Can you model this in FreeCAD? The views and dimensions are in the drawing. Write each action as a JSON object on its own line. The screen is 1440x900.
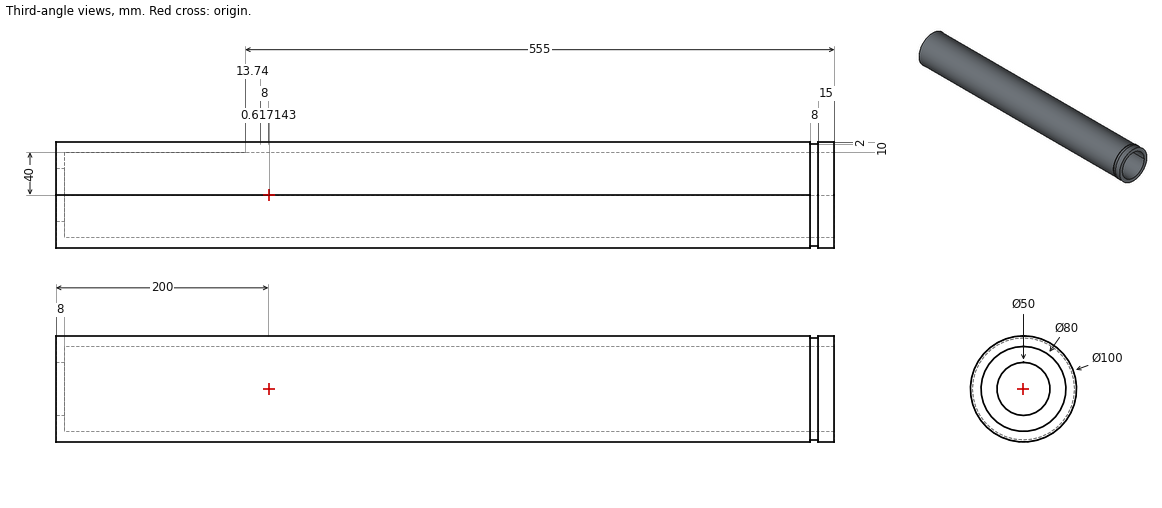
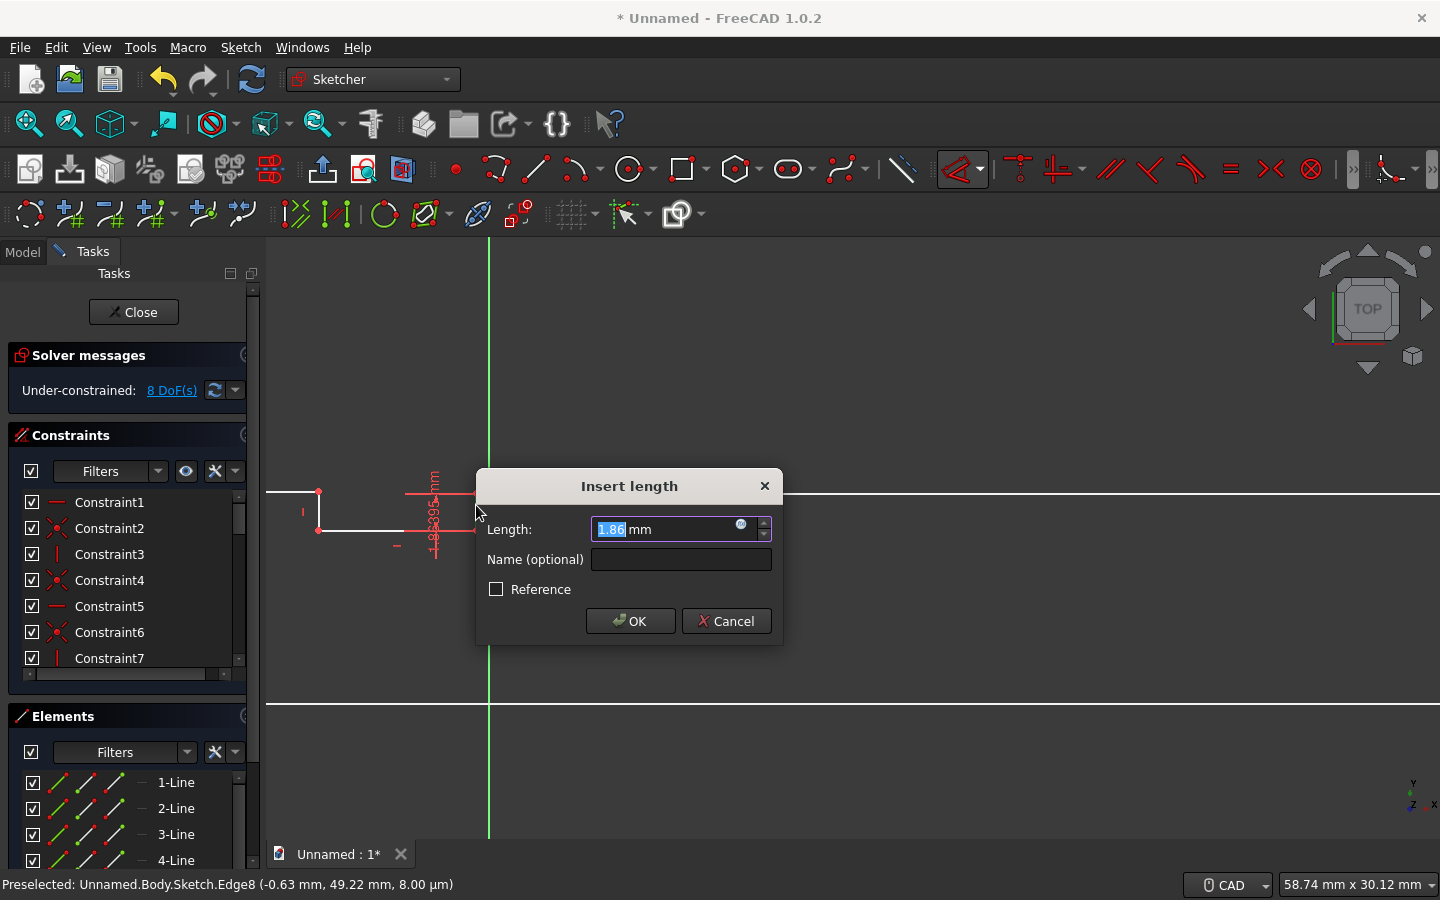
{"action": "type", "text": "2"}
{"action": "key", "text": "Return"}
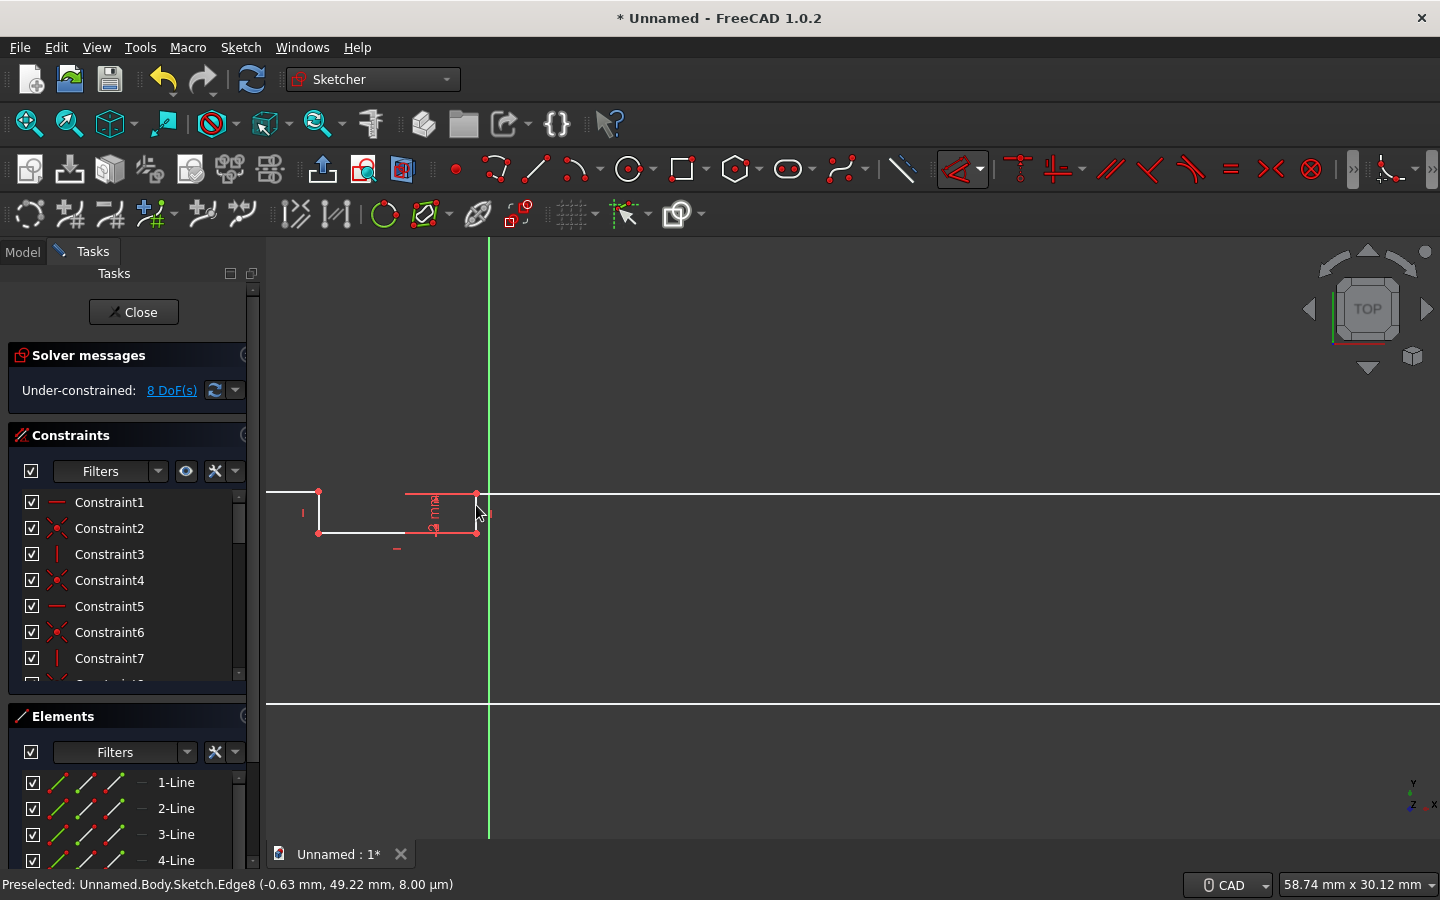
{"action": "scroll", "coordinate": [473, 509], "scroll_direction": "down", "scroll_amount": 14}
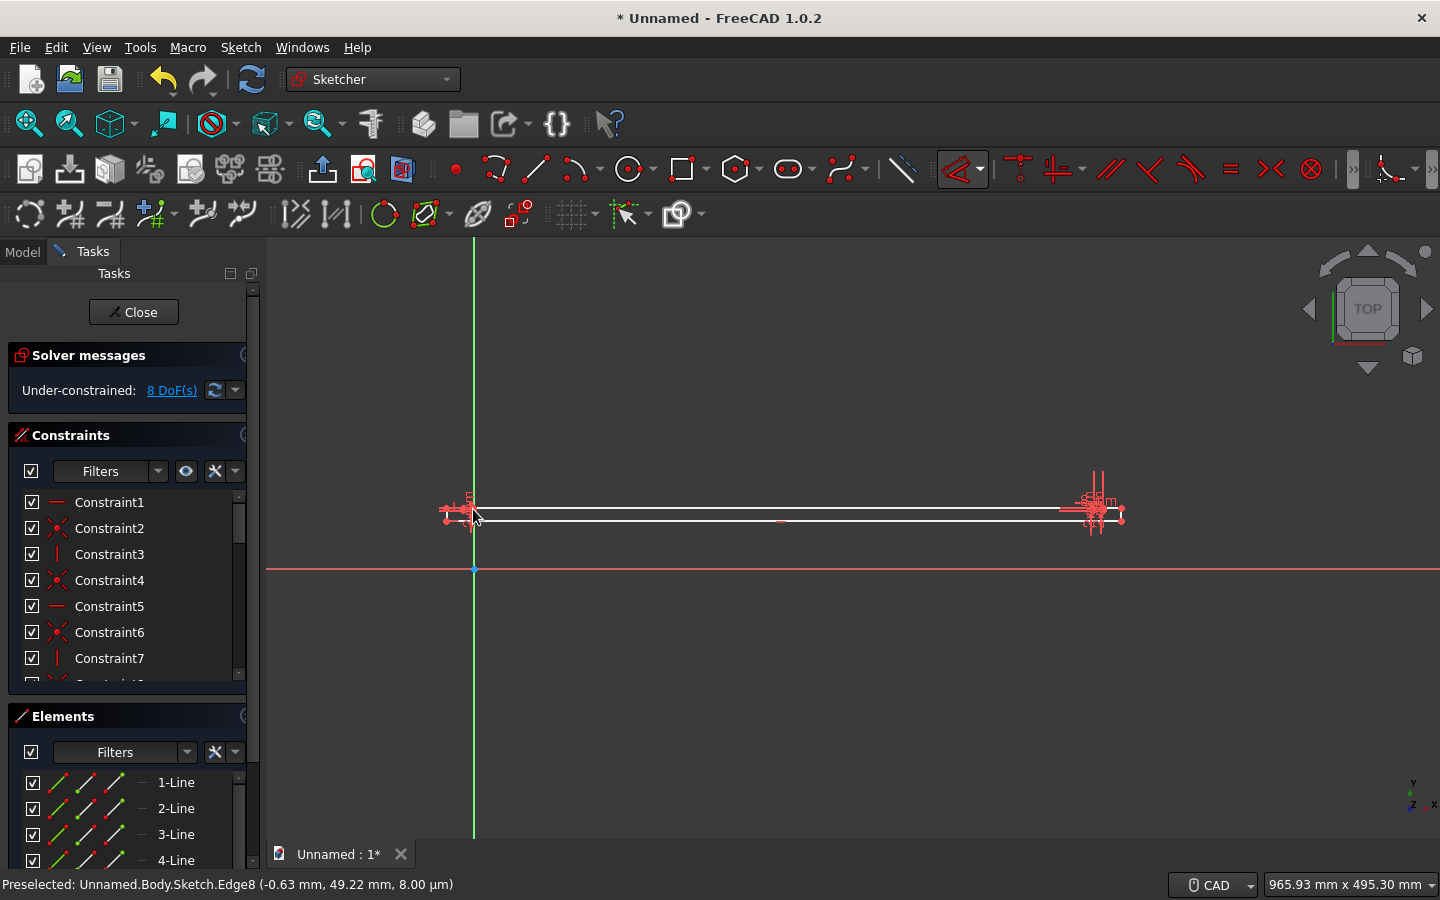
{"action": "scroll", "coordinate": [470, 511], "scroll_direction": "up", "scroll_amount": 8}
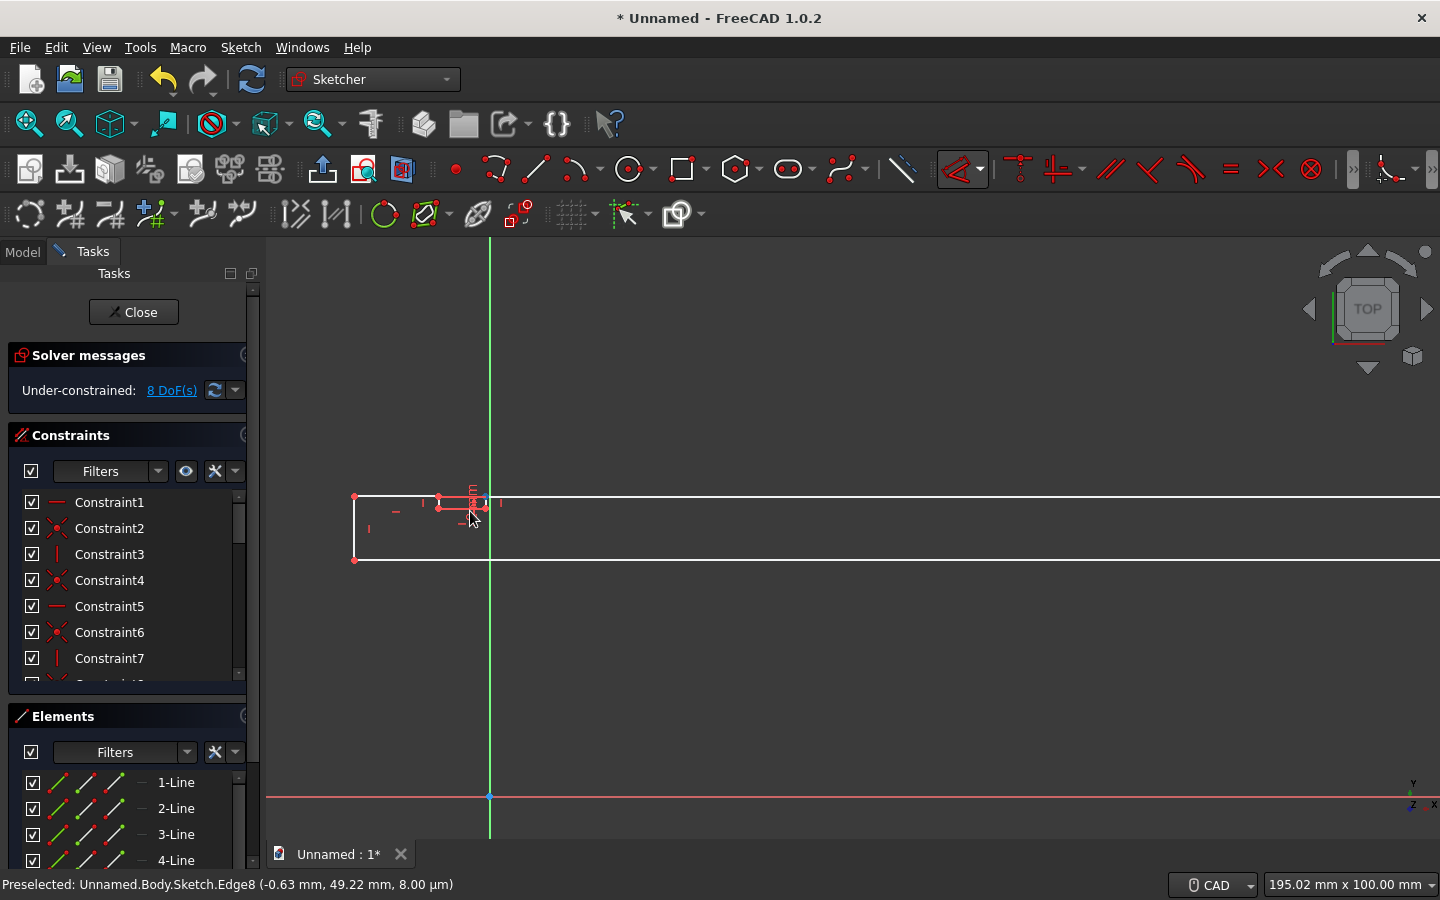
{"action": "left_click", "coordinate": [453, 509]}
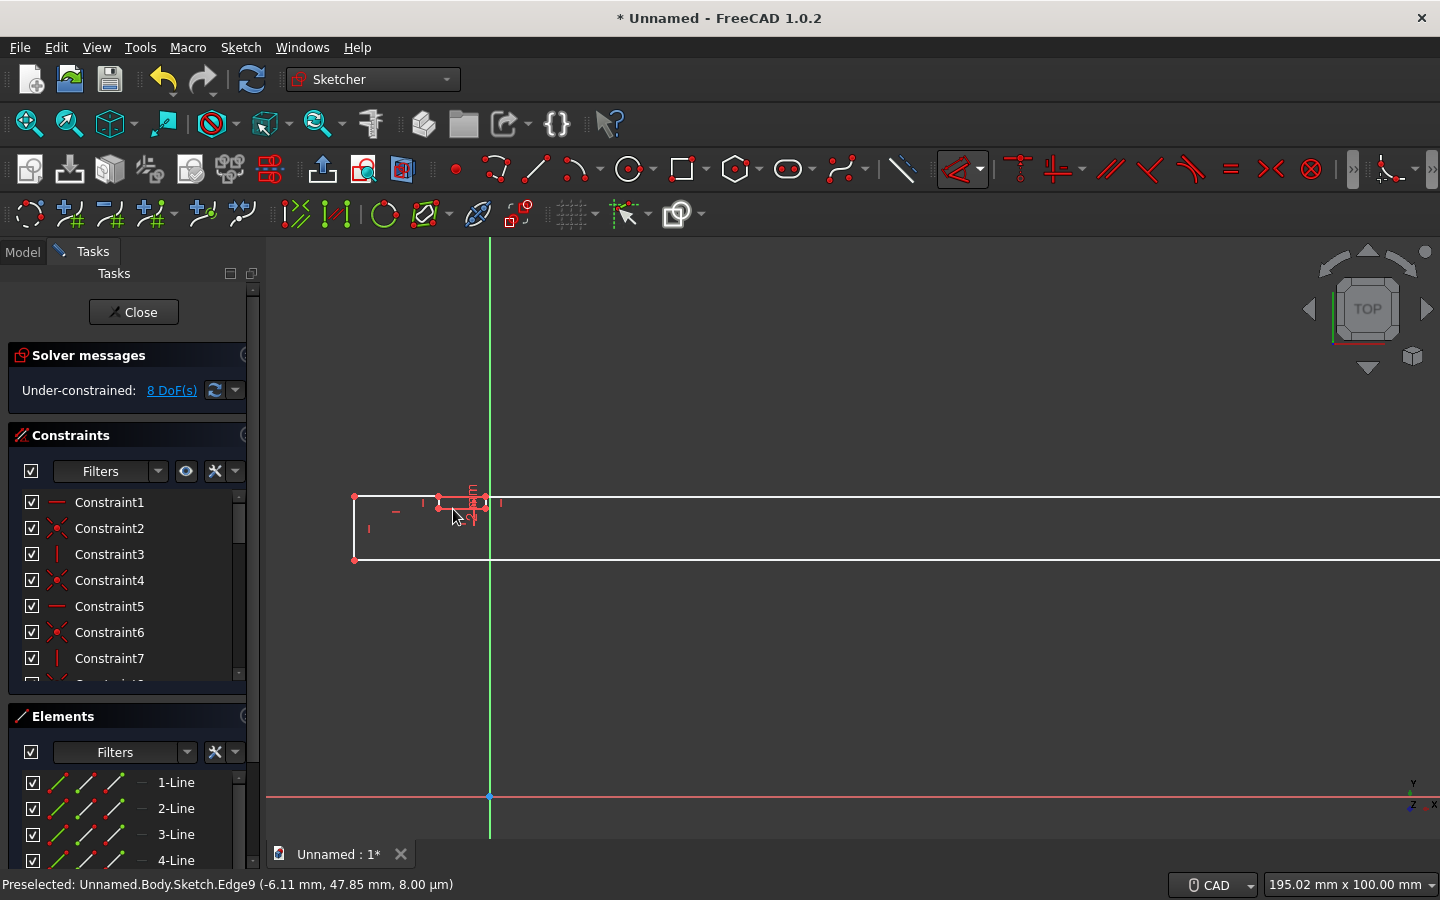
{"action": "key", "text": "l"}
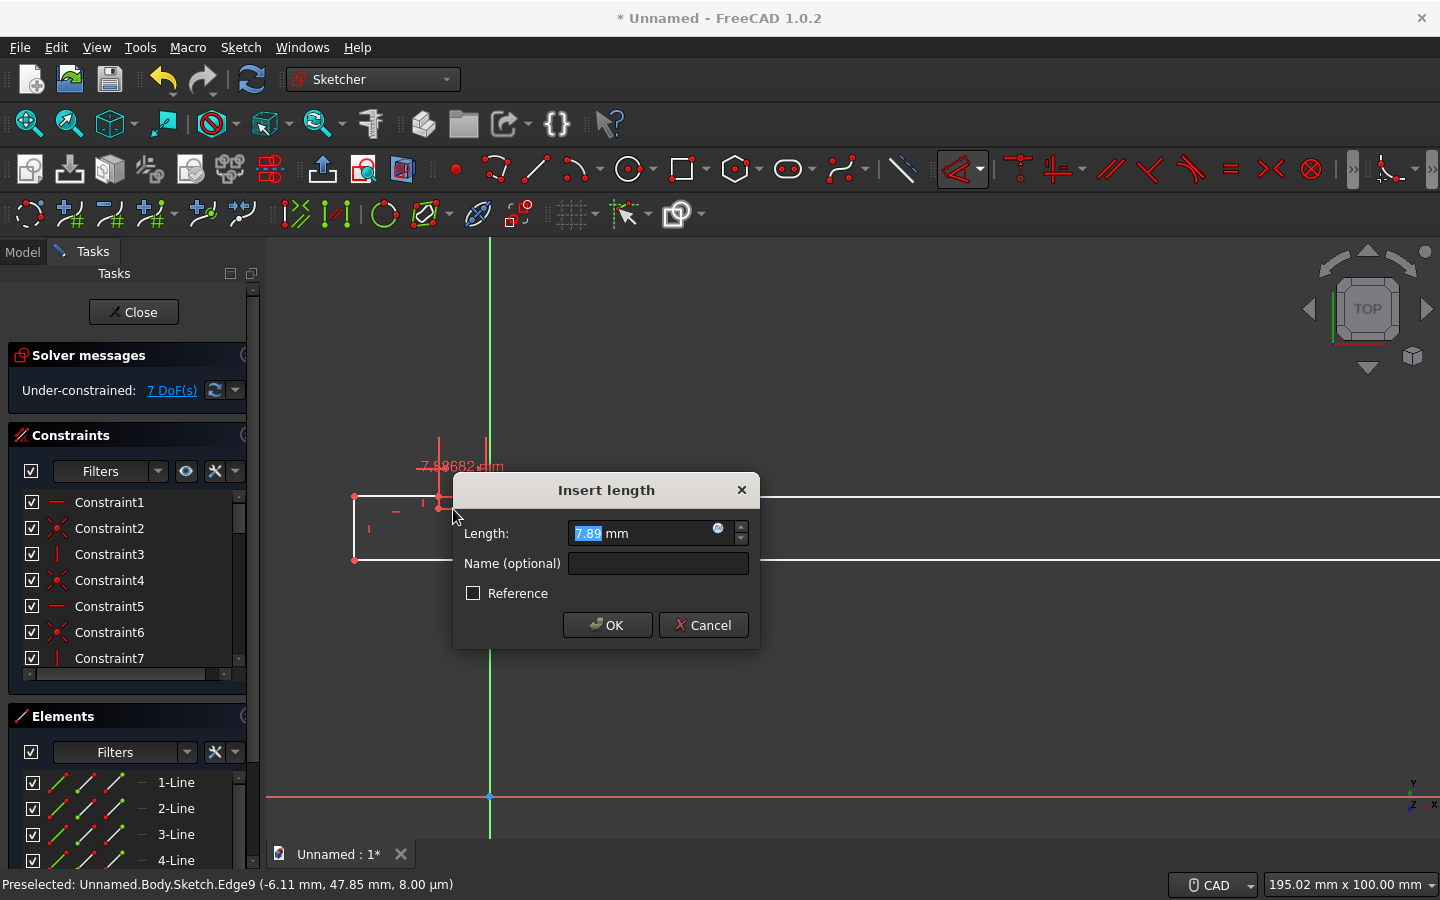
{"action": "type", "text": "8"}
{"action": "key", "text": "Return"}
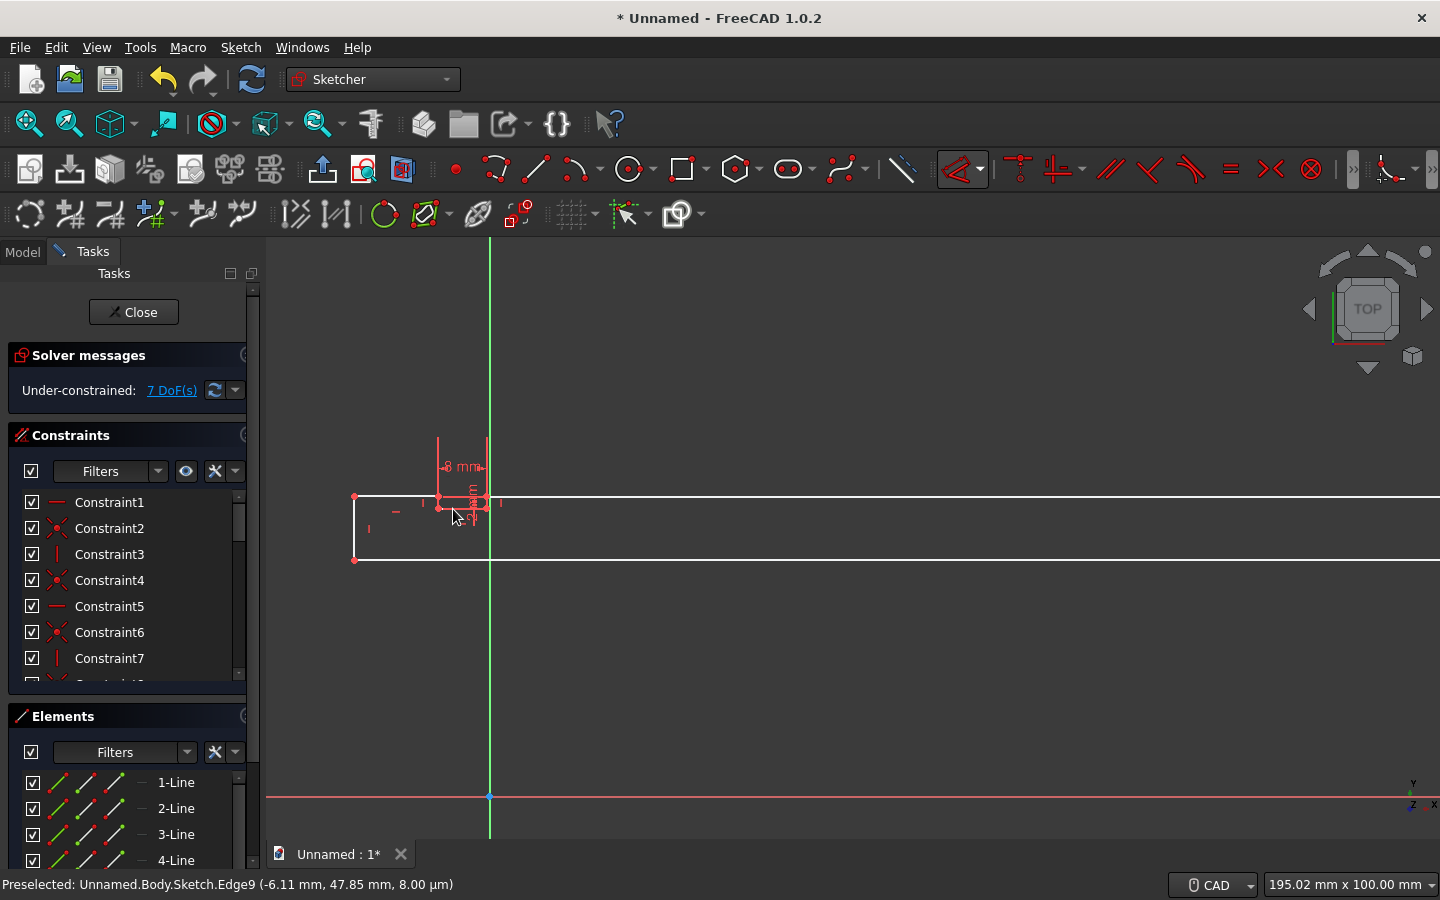
{"action": "scroll", "coordinate": [438, 502], "scroll_direction": "up", "scroll_amount": 6}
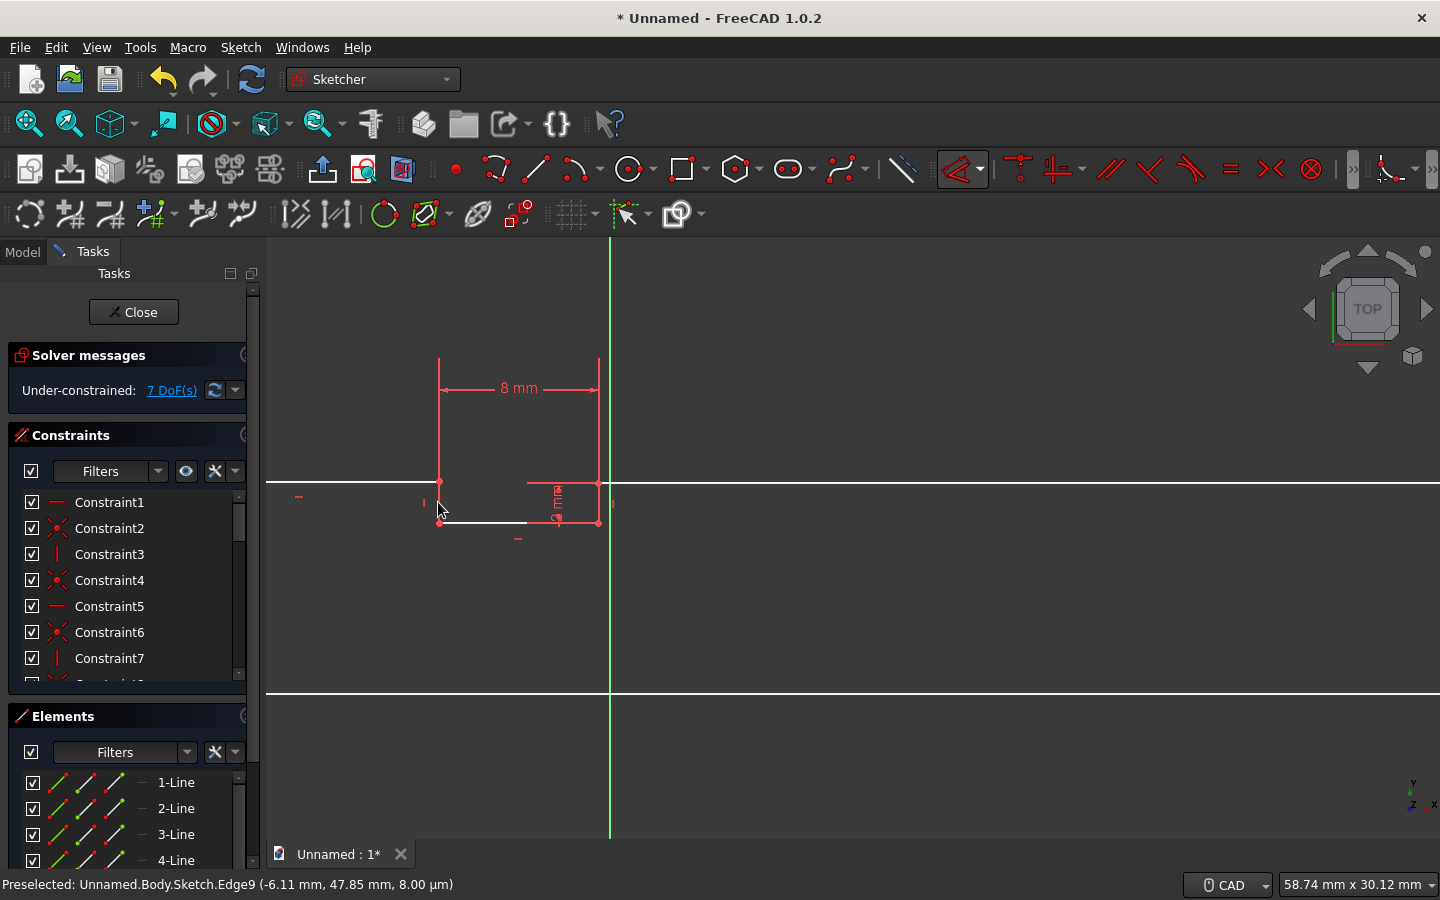
{"action": "left_click", "coordinate": [439, 503]}